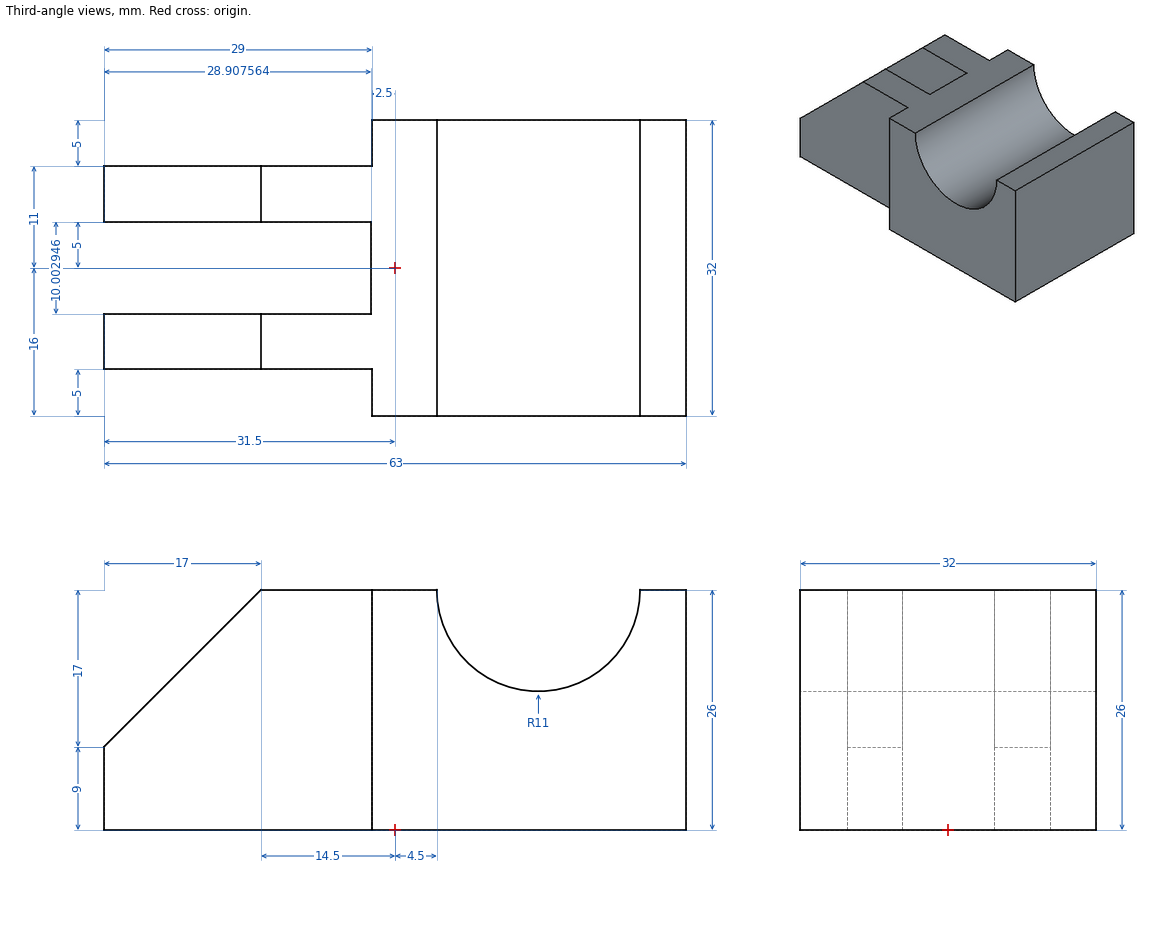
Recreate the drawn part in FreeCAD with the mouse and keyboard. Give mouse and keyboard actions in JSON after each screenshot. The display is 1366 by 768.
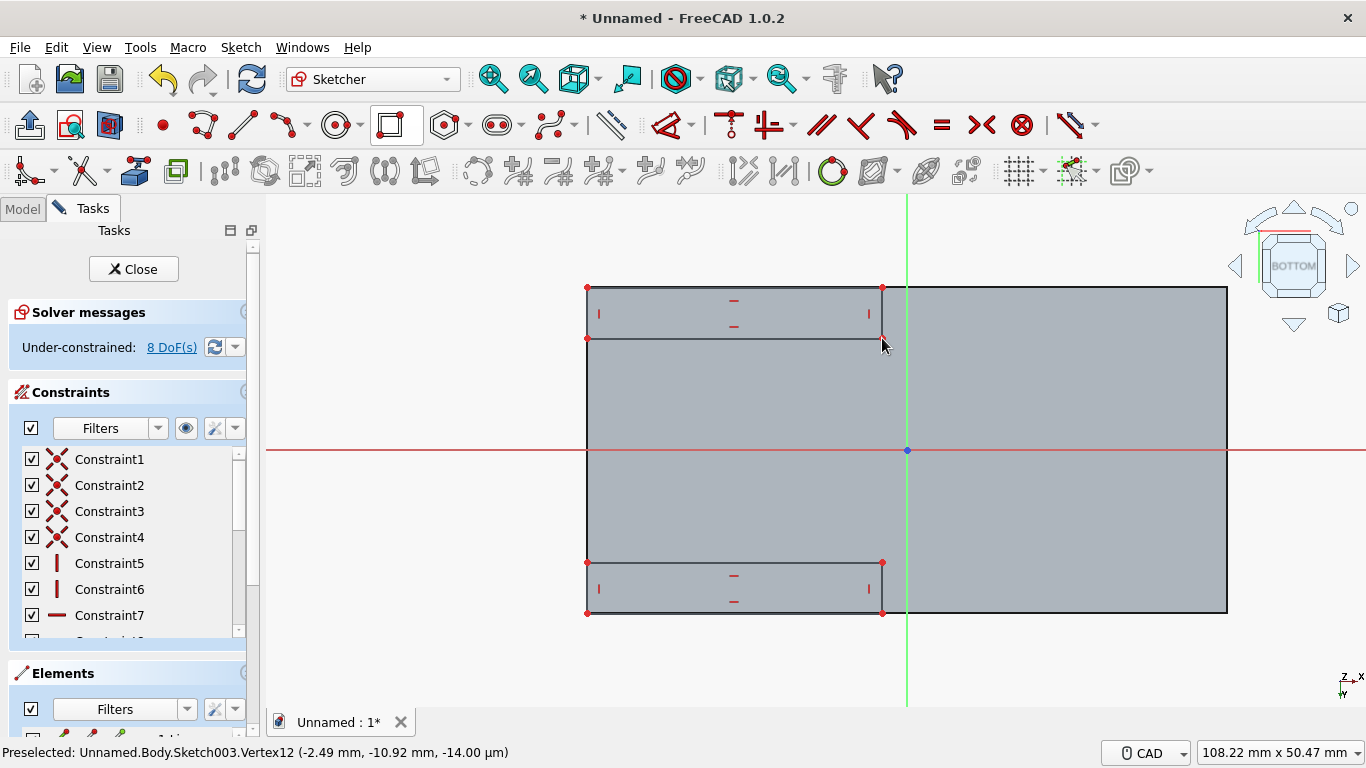
{"action": "left_click", "coordinate": [666, 126]}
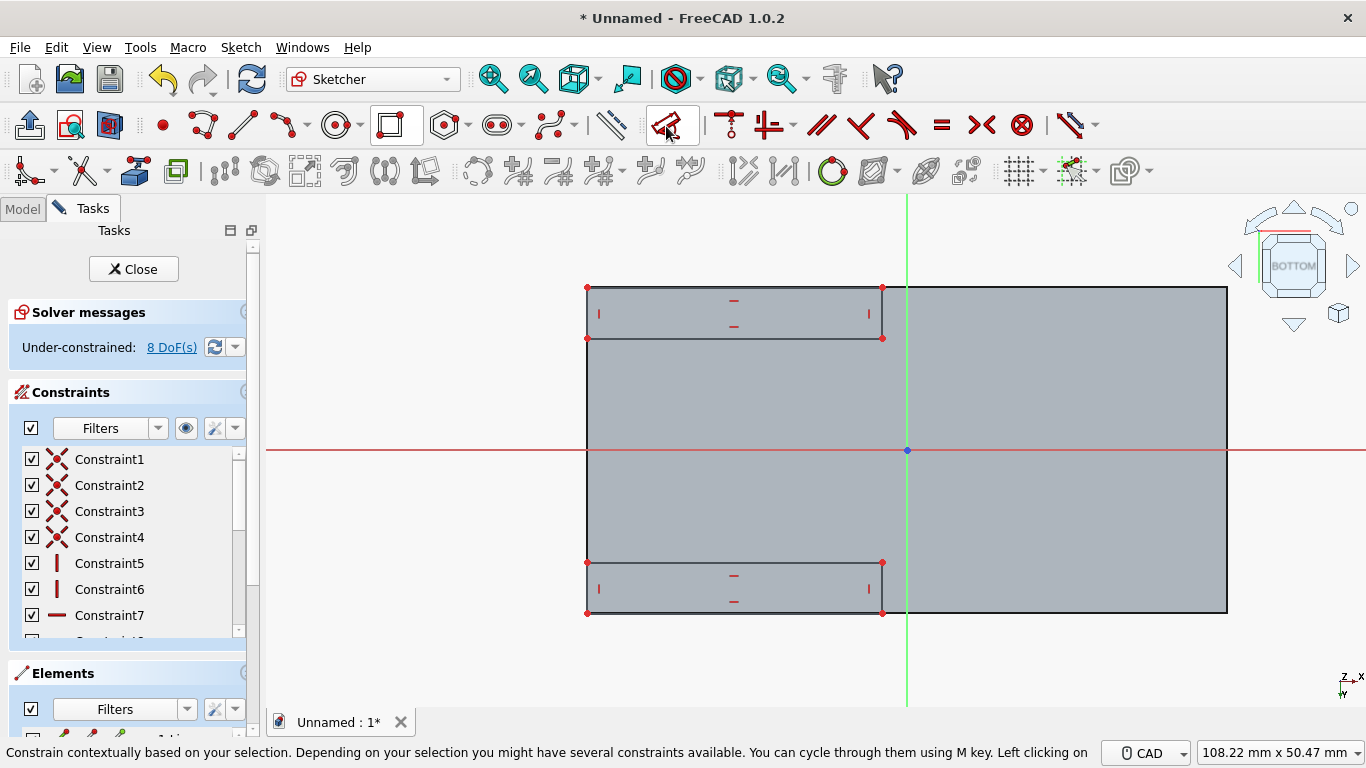
{"action": "left_click", "coordinate": [587, 578]}
{"action": "left_click", "coordinate": [553, 588]}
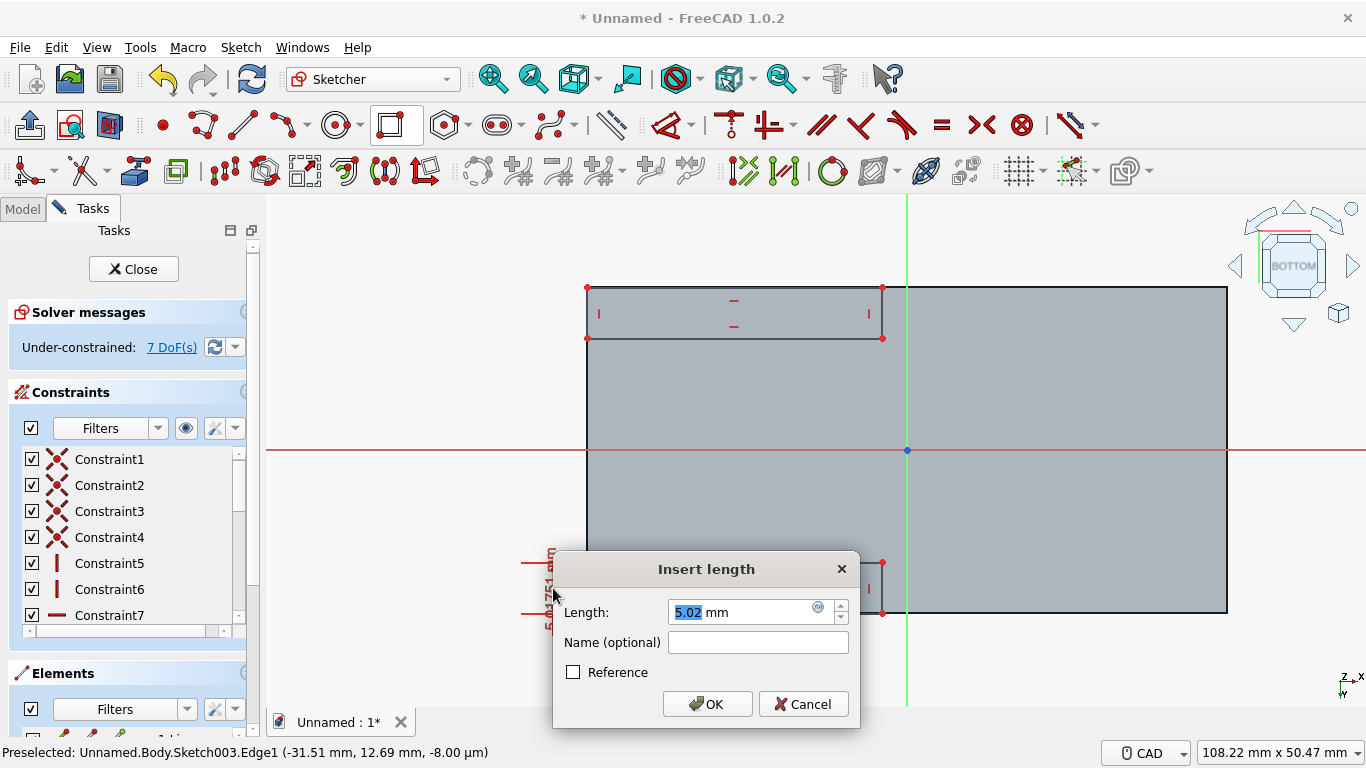
{"action": "type", "text": "5"}
{"action": "key", "text": "Return"}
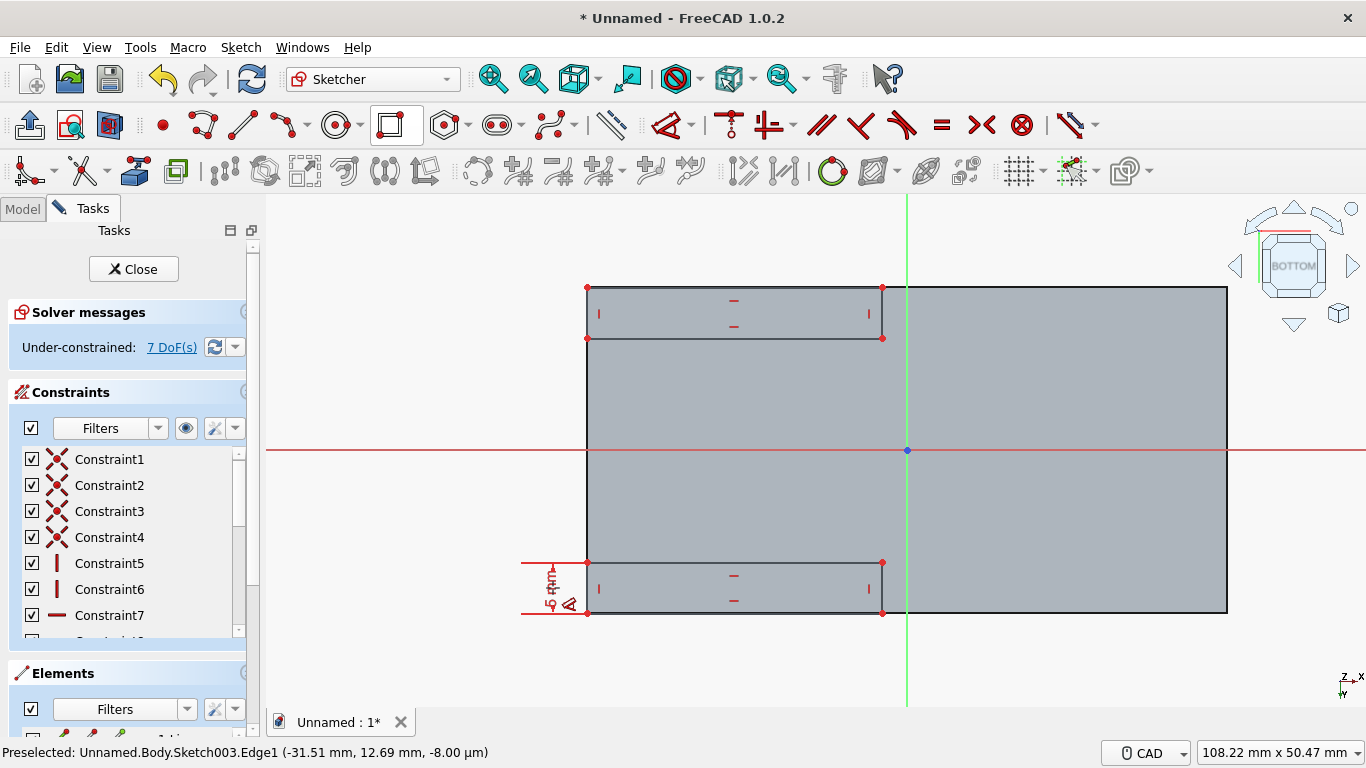
{"action": "left_click", "coordinate": [587, 303]}
{"action": "left_click", "coordinate": [553, 314]}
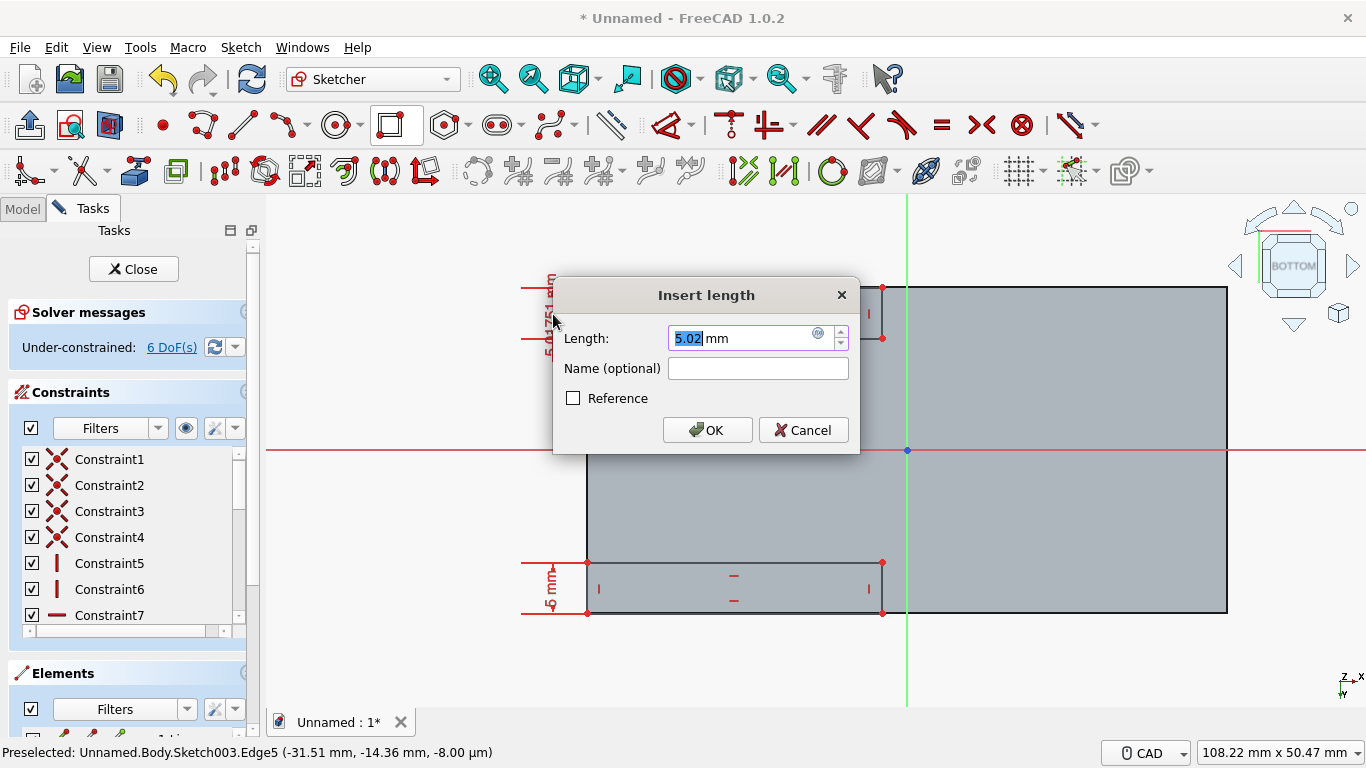
{"action": "type", "text": "5"}
{"action": "key", "text": "Return"}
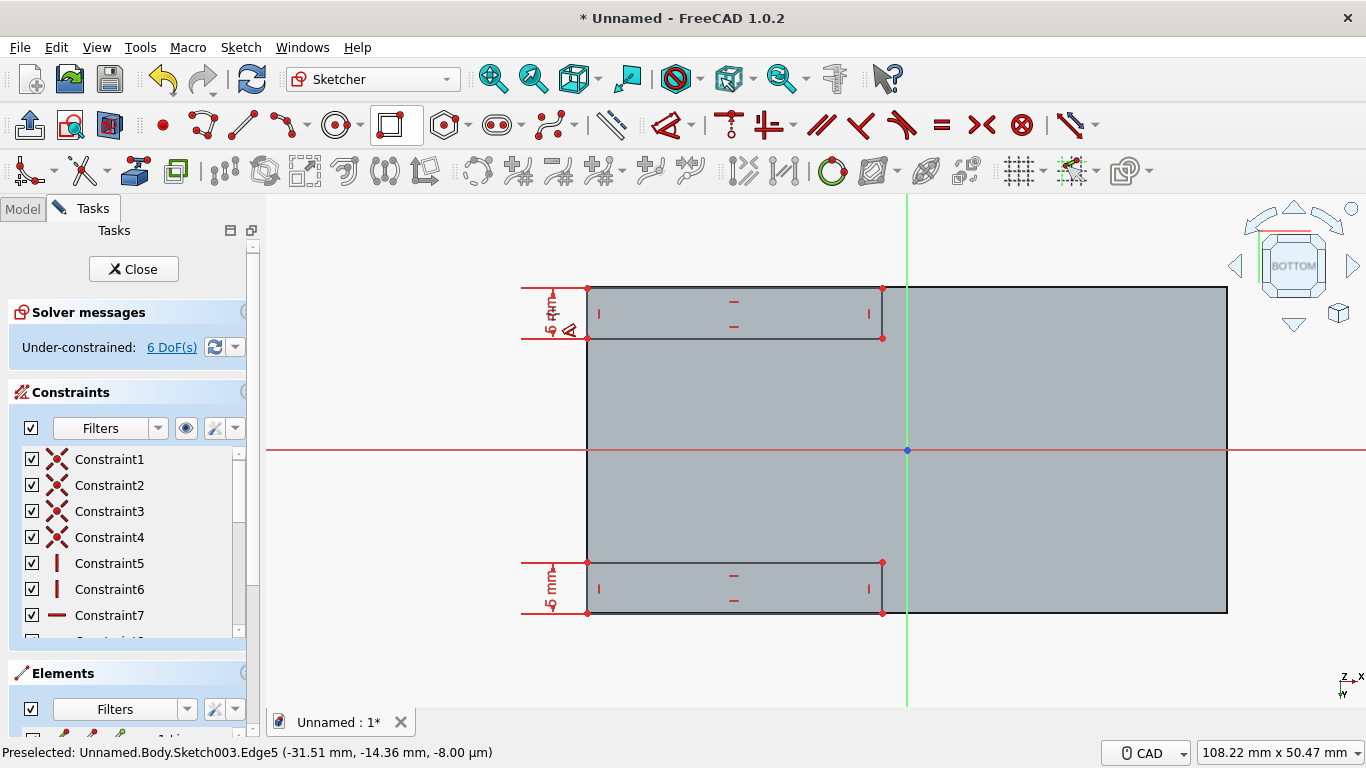
{"action": "left_click", "coordinate": [675, 614]}
{"action": "left_click", "coordinate": [734, 648]}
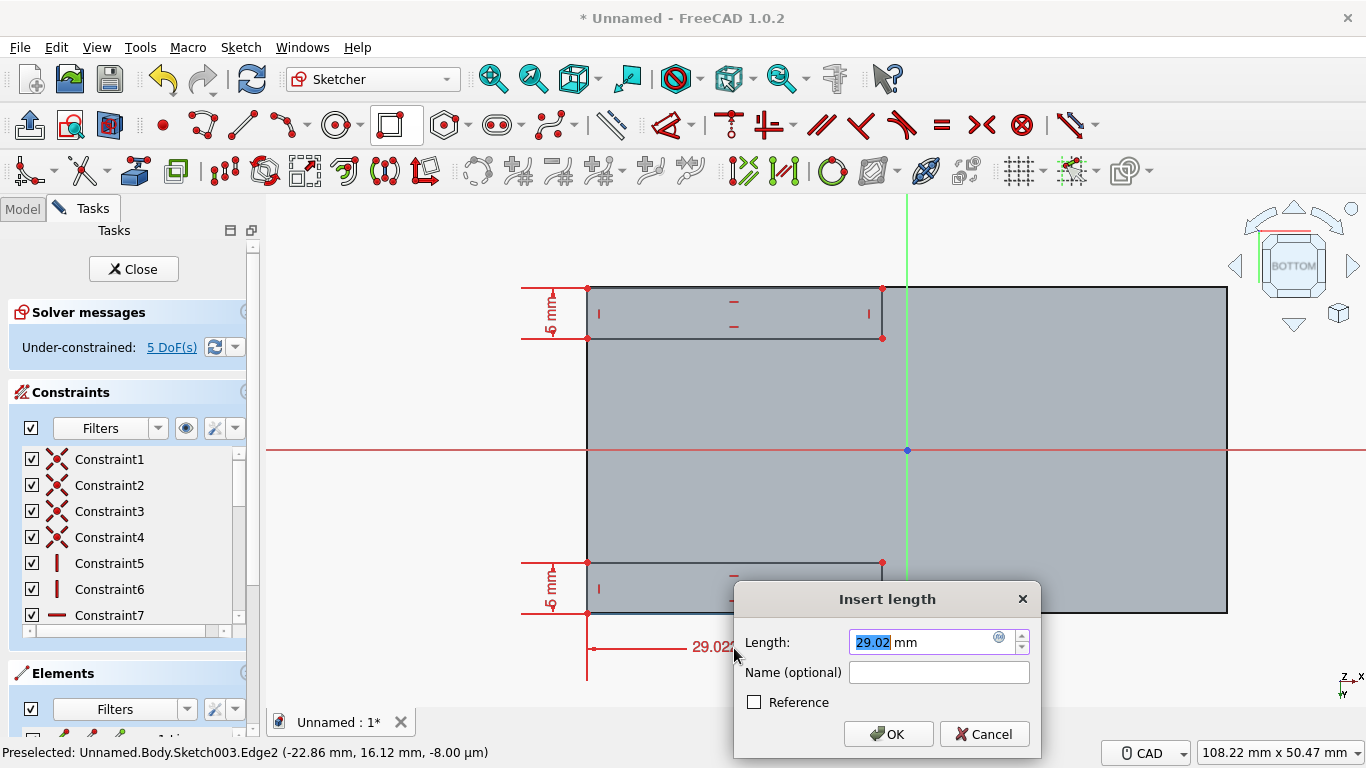
{"action": "type", "text": "29"}
{"action": "key", "text": "Return"}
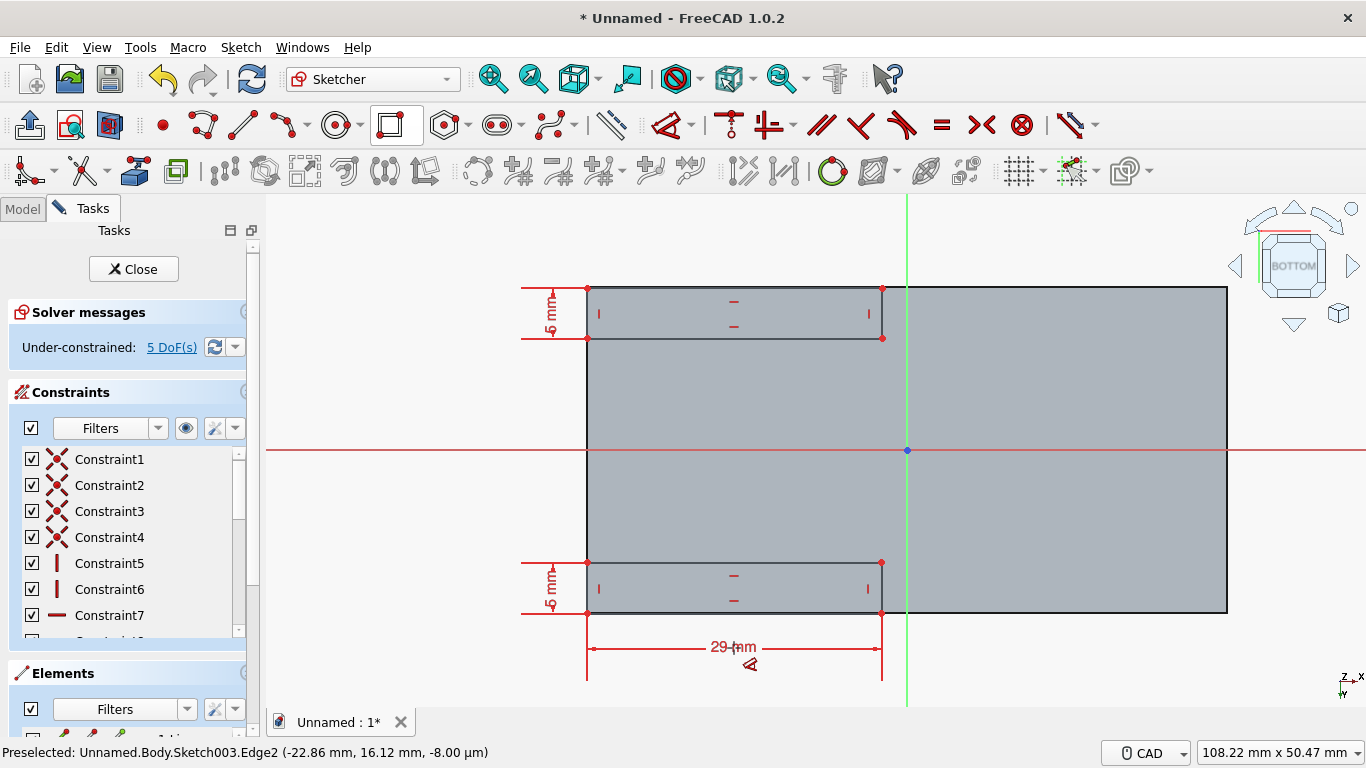
{"action": "left_click", "coordinate": [675, 339]}
{"action": "left_click", "coordinate": [734, 305]}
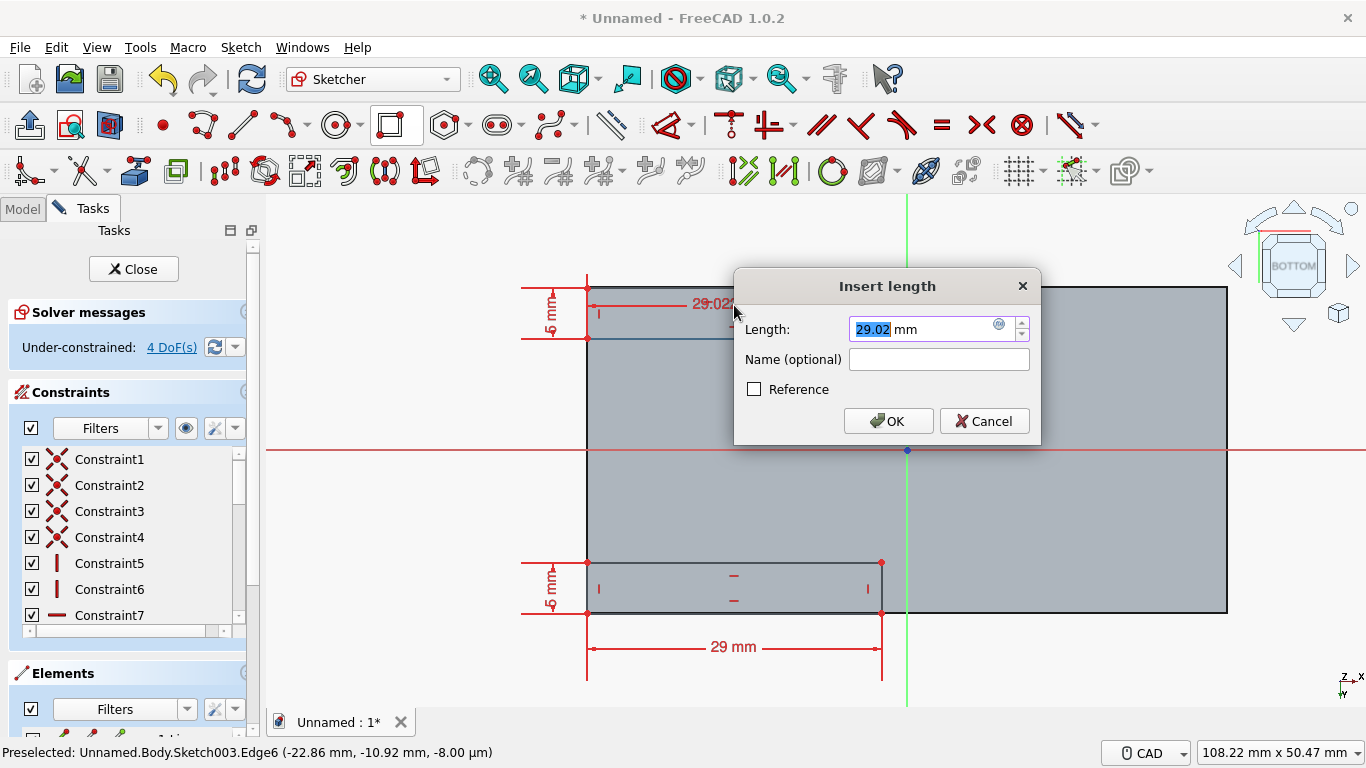
{"action": "type", "text": "29"}
{"action": "key", "text": "Return"}